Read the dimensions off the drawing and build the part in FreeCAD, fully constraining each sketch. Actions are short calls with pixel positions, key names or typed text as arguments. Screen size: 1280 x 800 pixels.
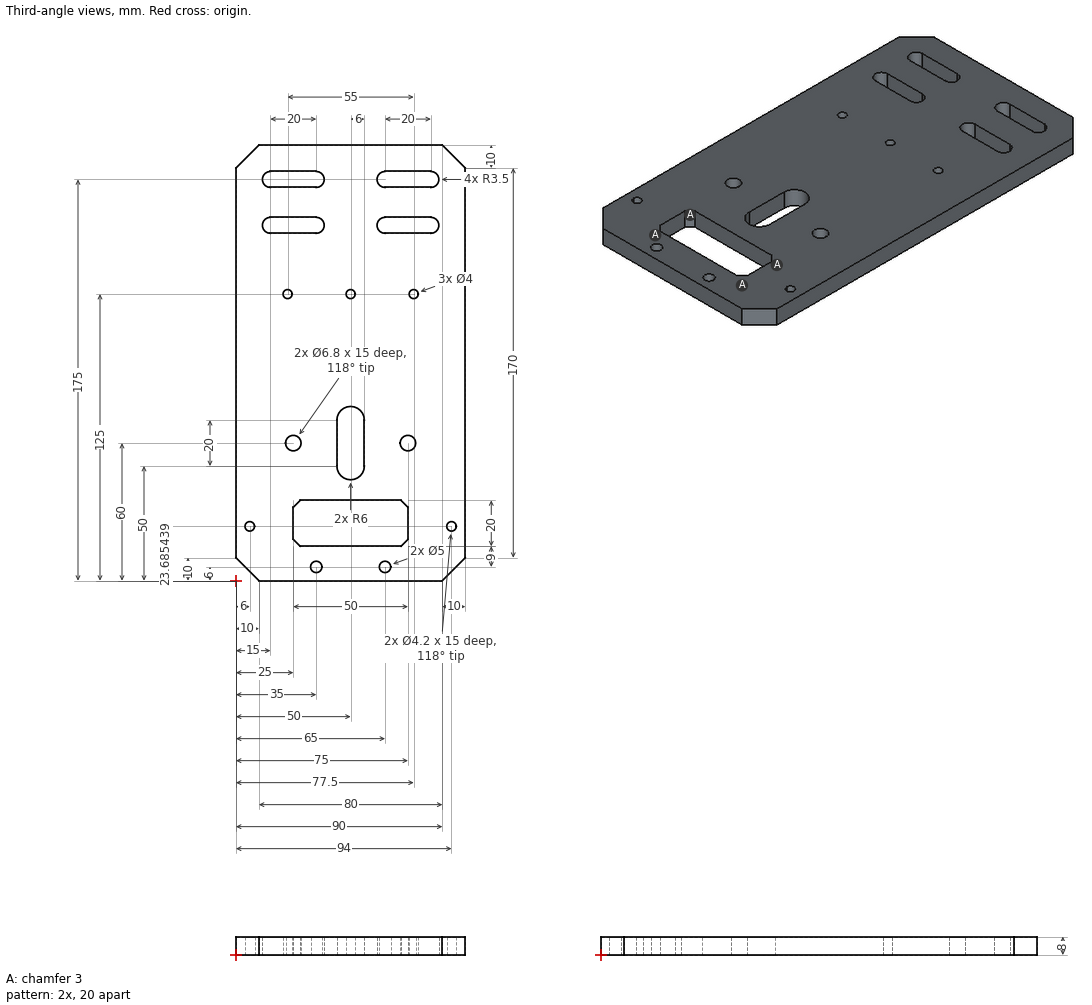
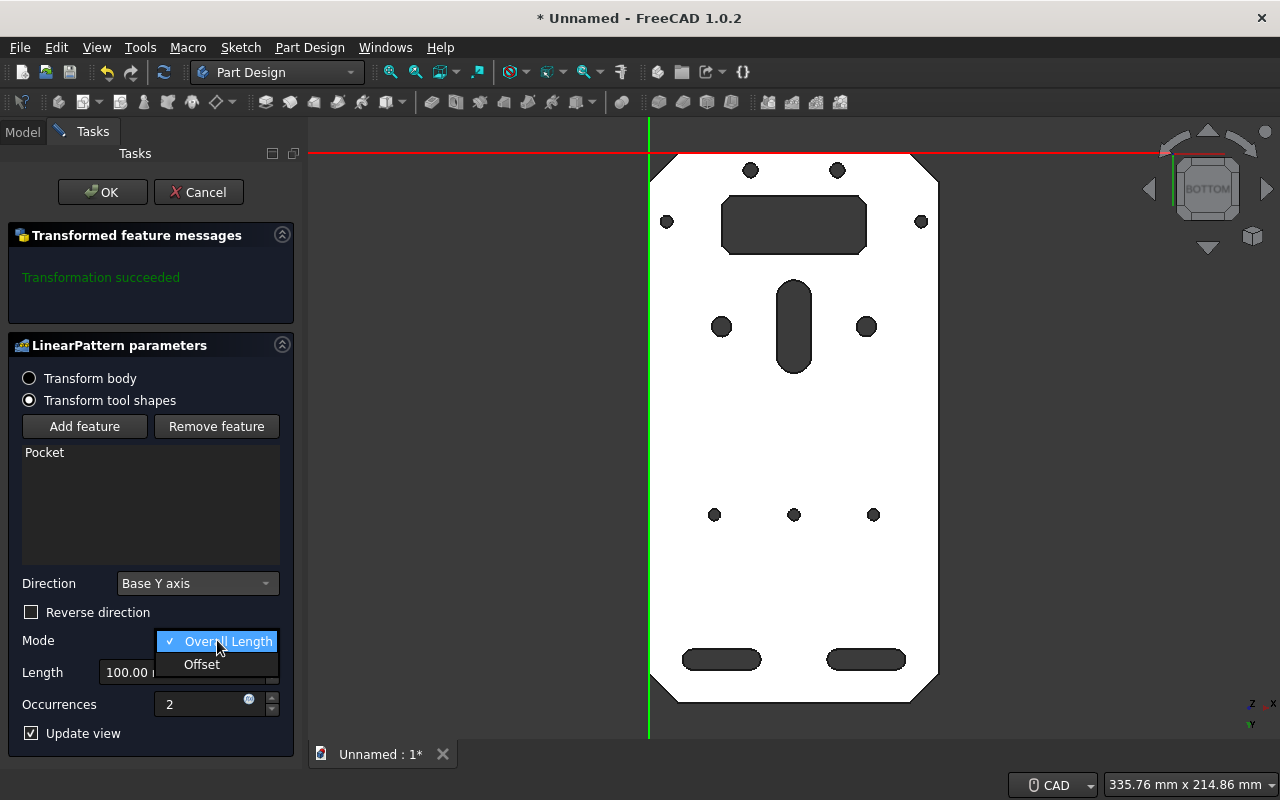
click(216, 664)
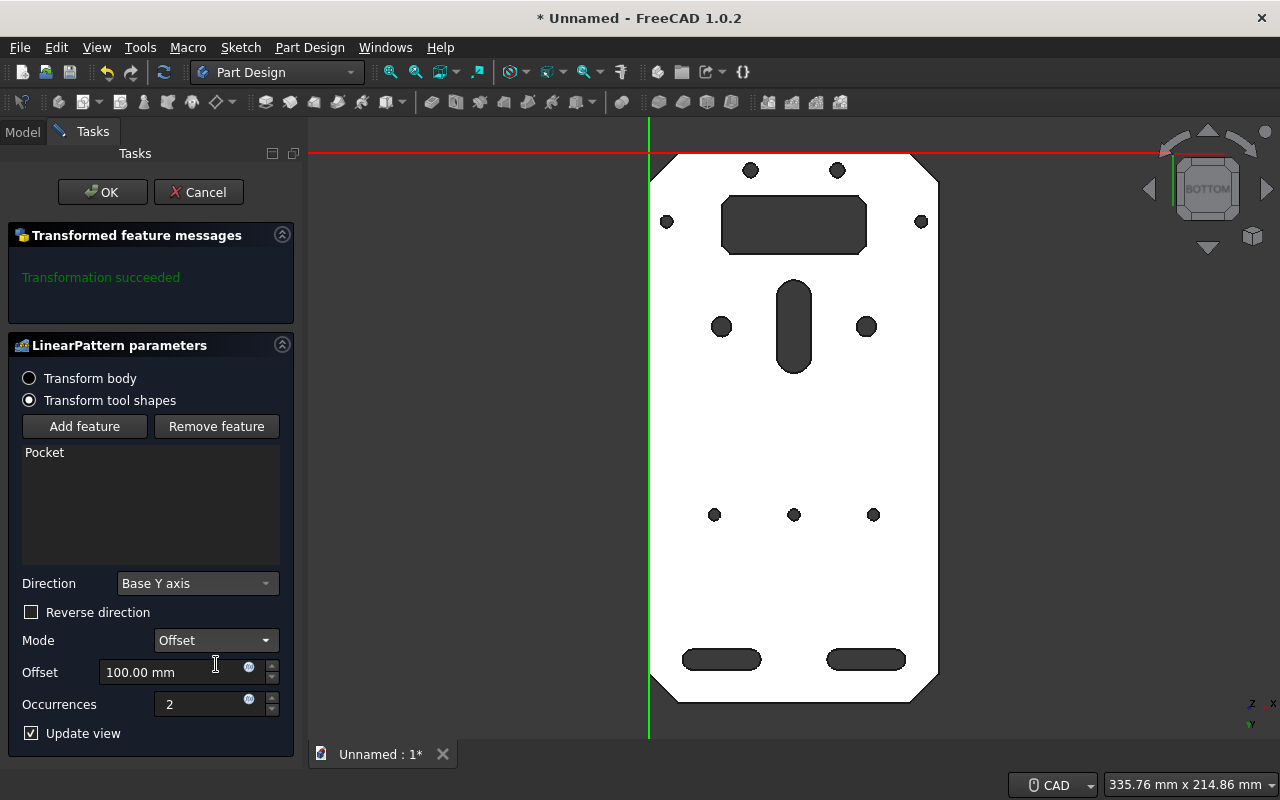
triple_click(182, 672)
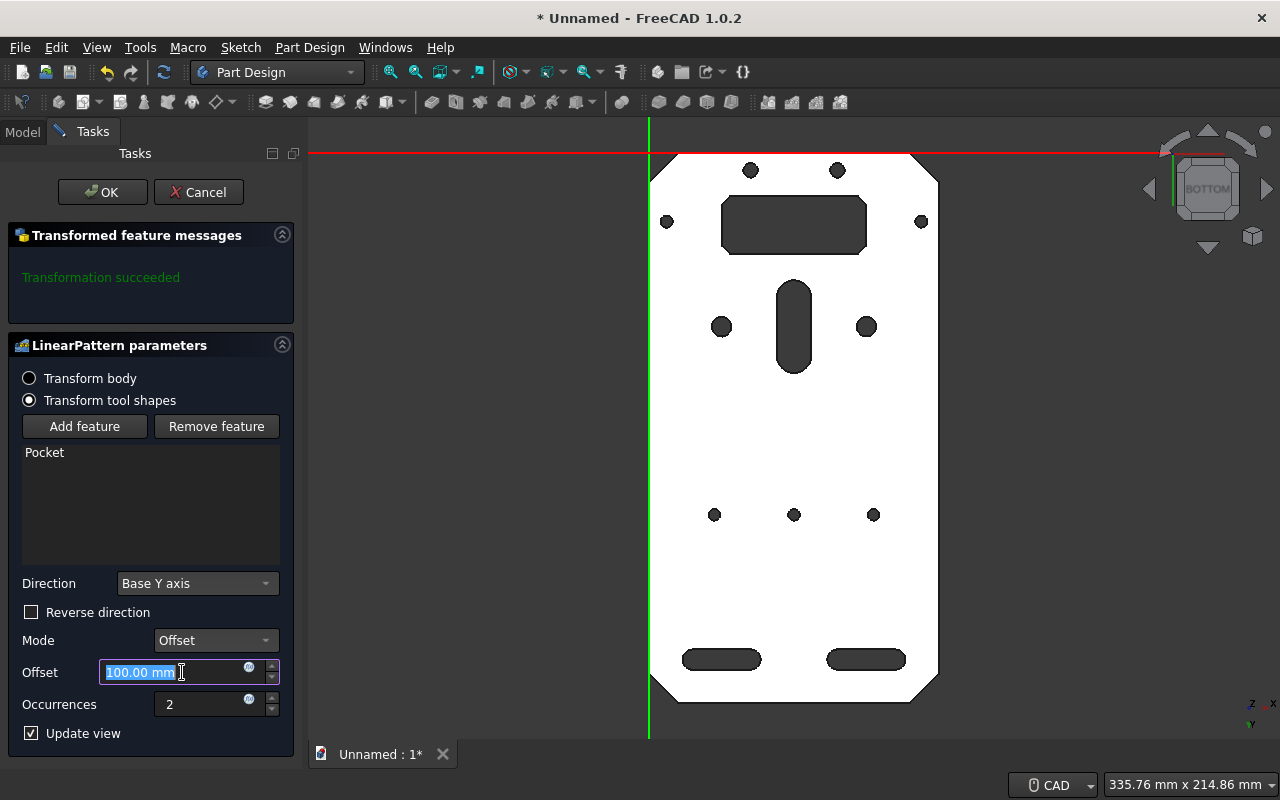
text(20)
key(Tab)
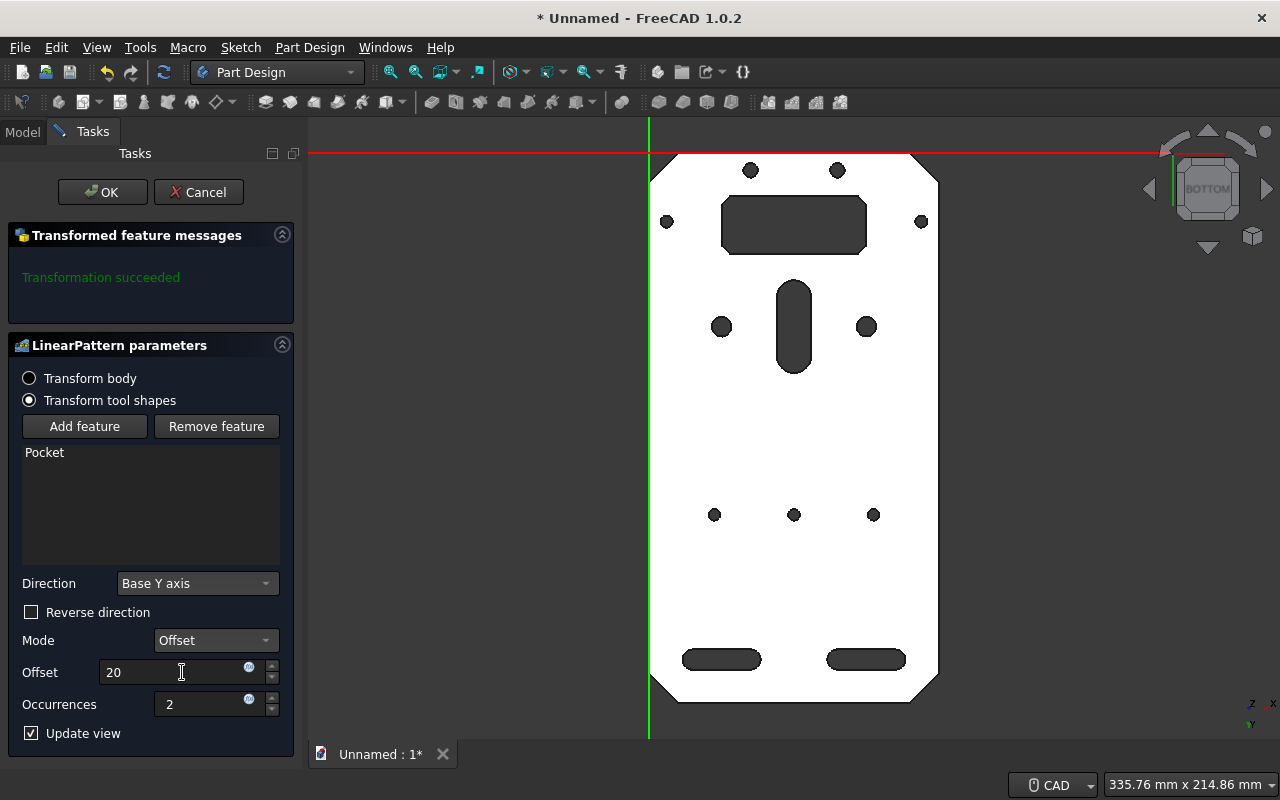
triple_click(209, 704)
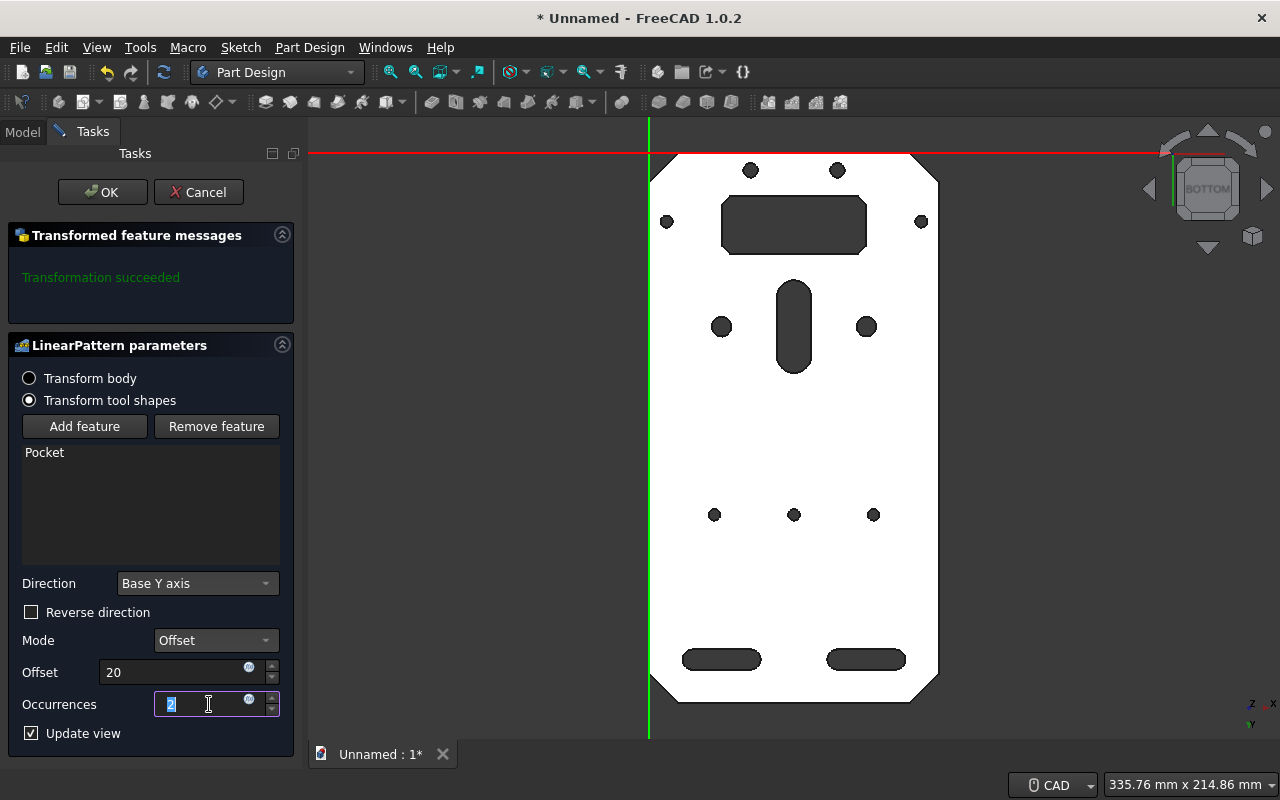
text(2)
key(Tab)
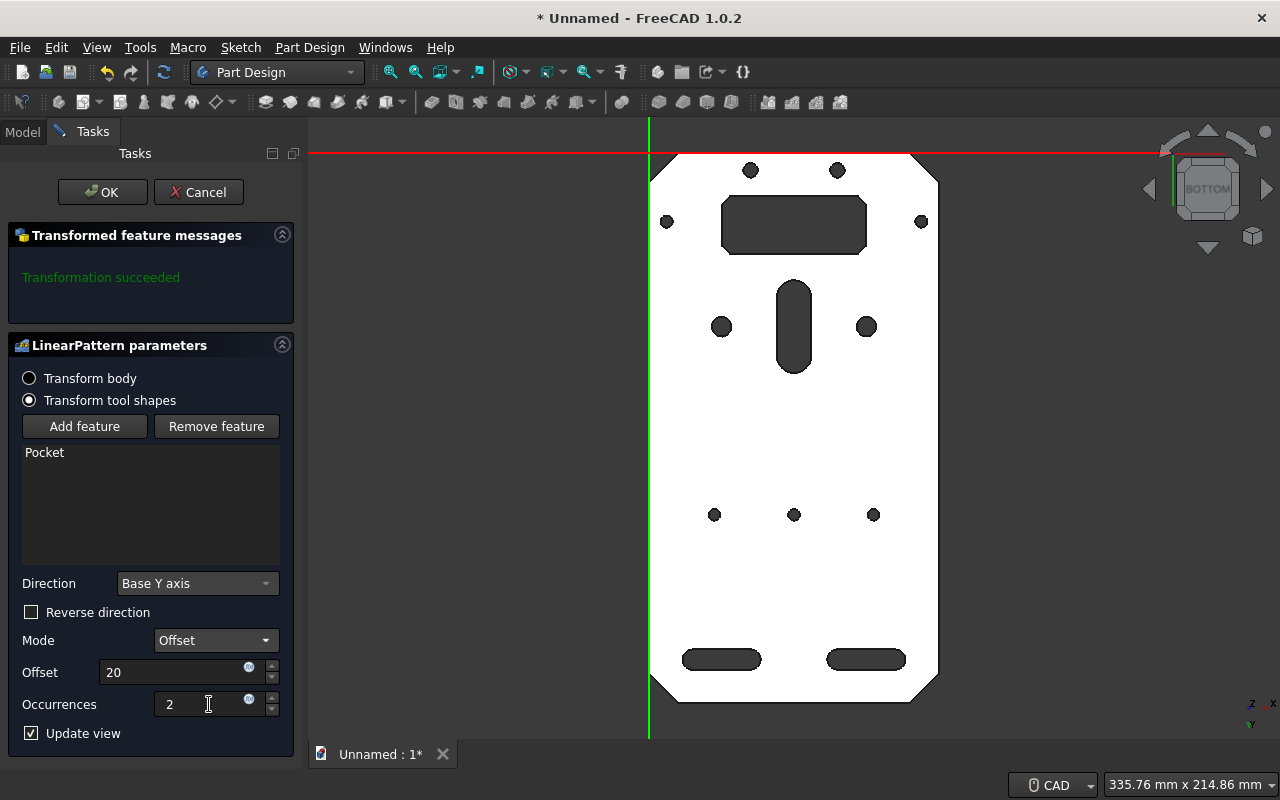
click(30, 612)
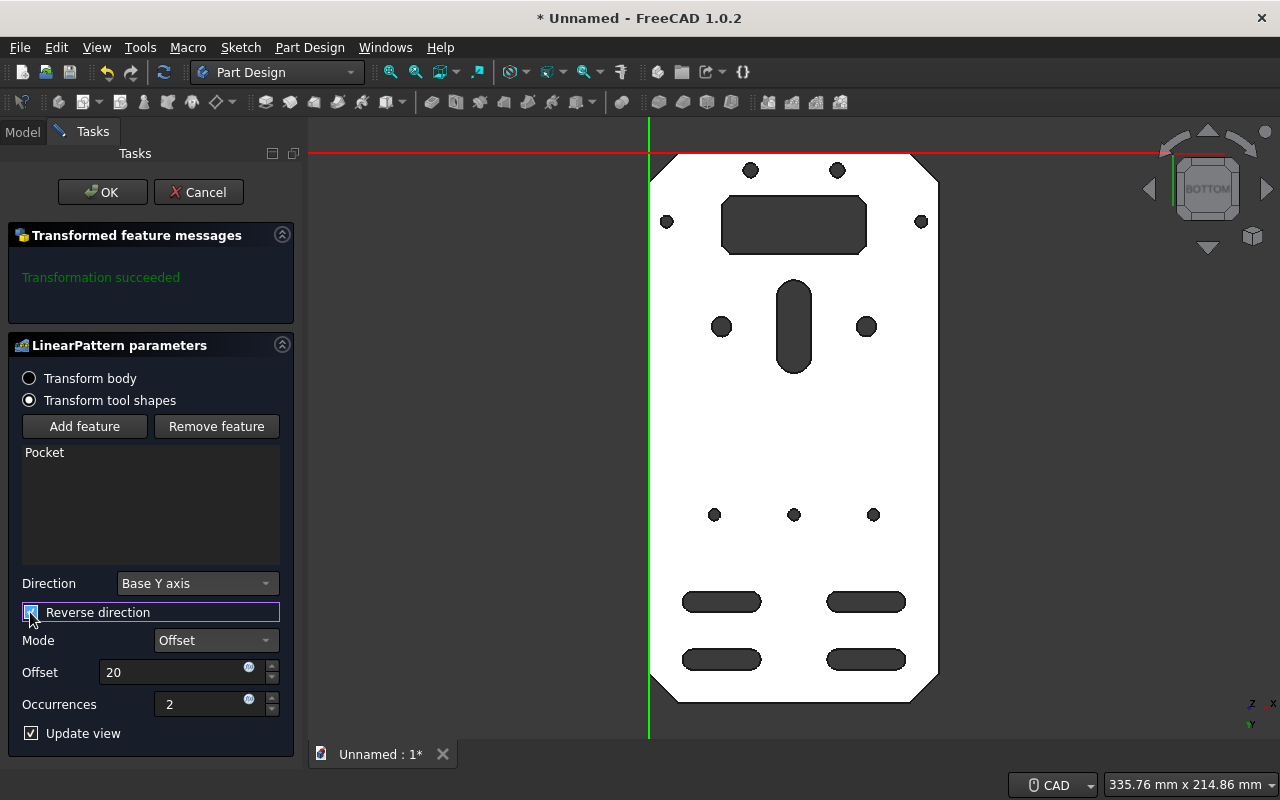
click(103, 192)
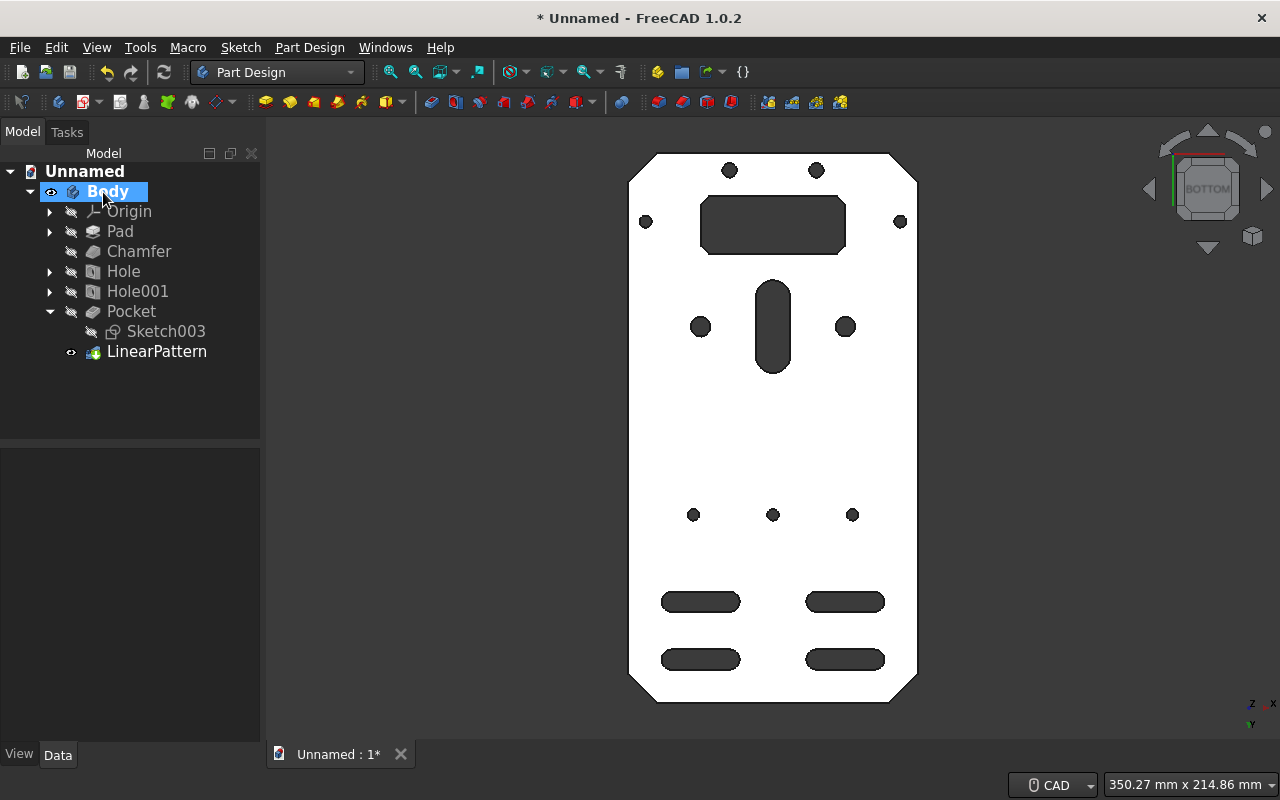
key(0)